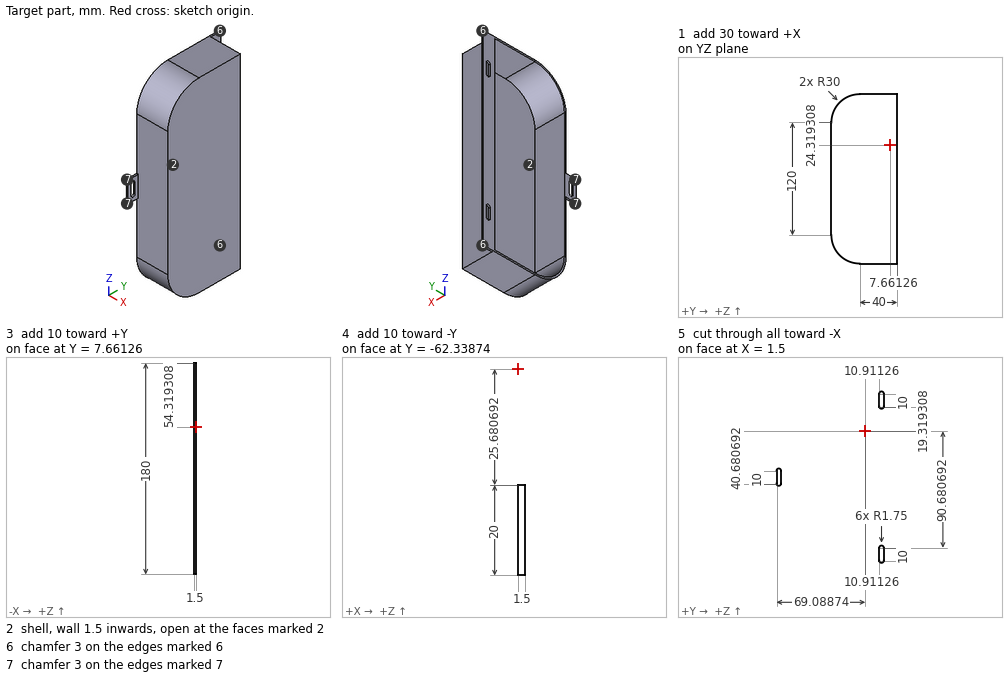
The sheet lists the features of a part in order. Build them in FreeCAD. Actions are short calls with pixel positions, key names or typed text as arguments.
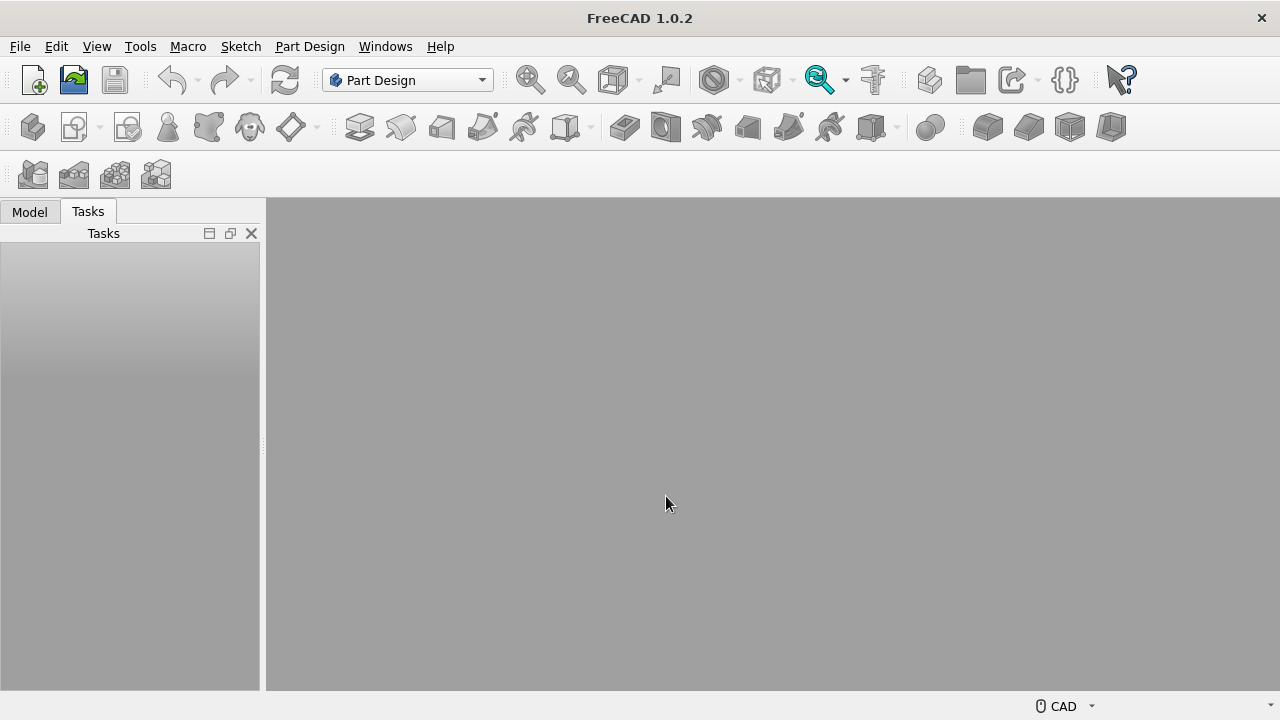
click(33, 80)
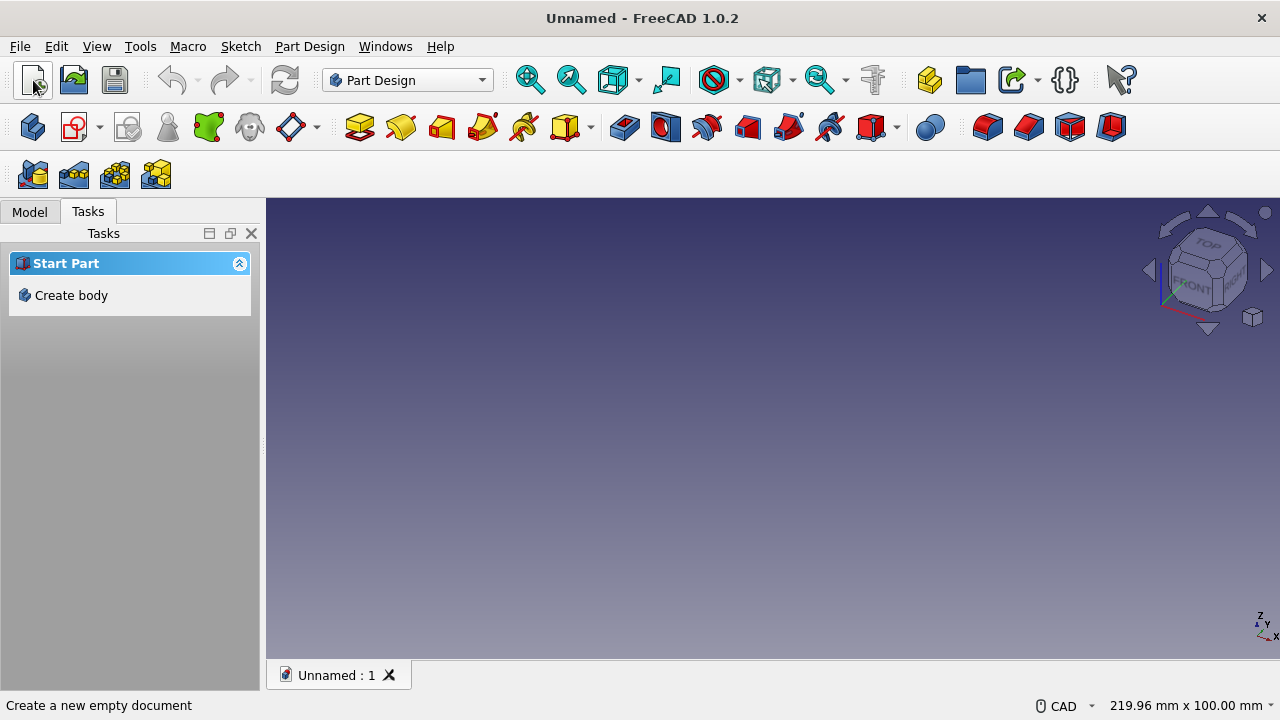
click(74, 128)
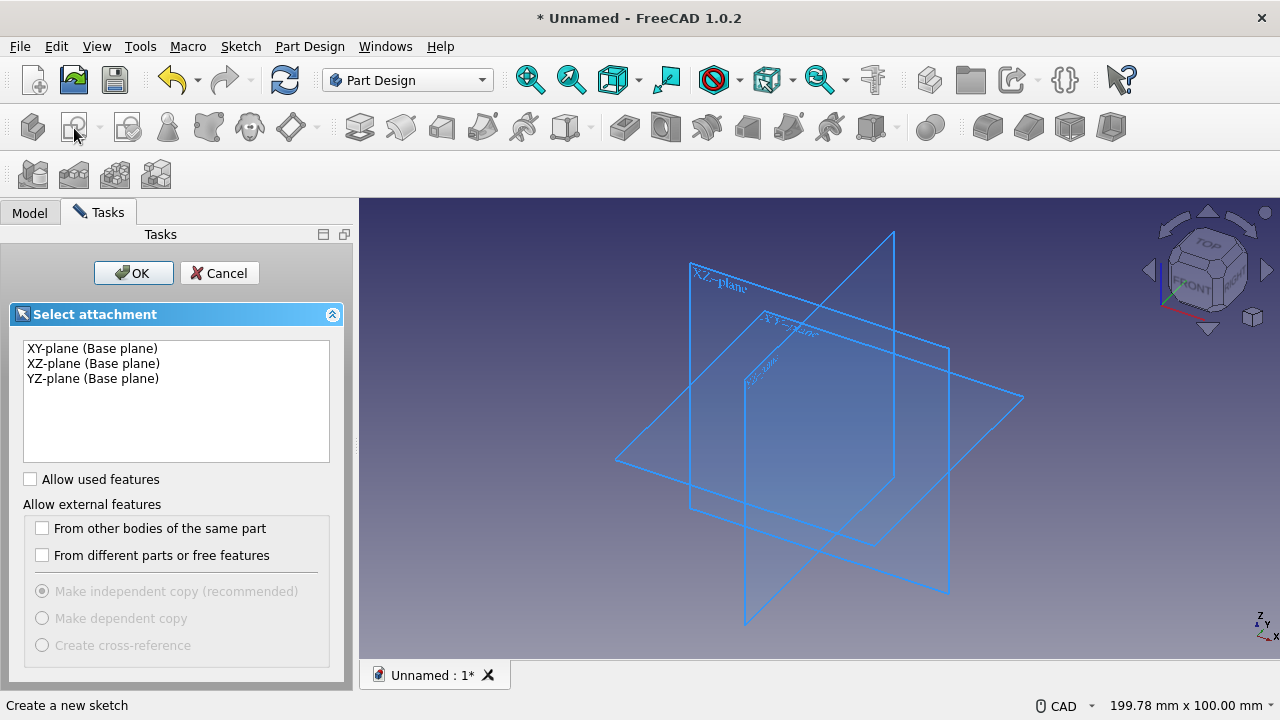
click(84, 378)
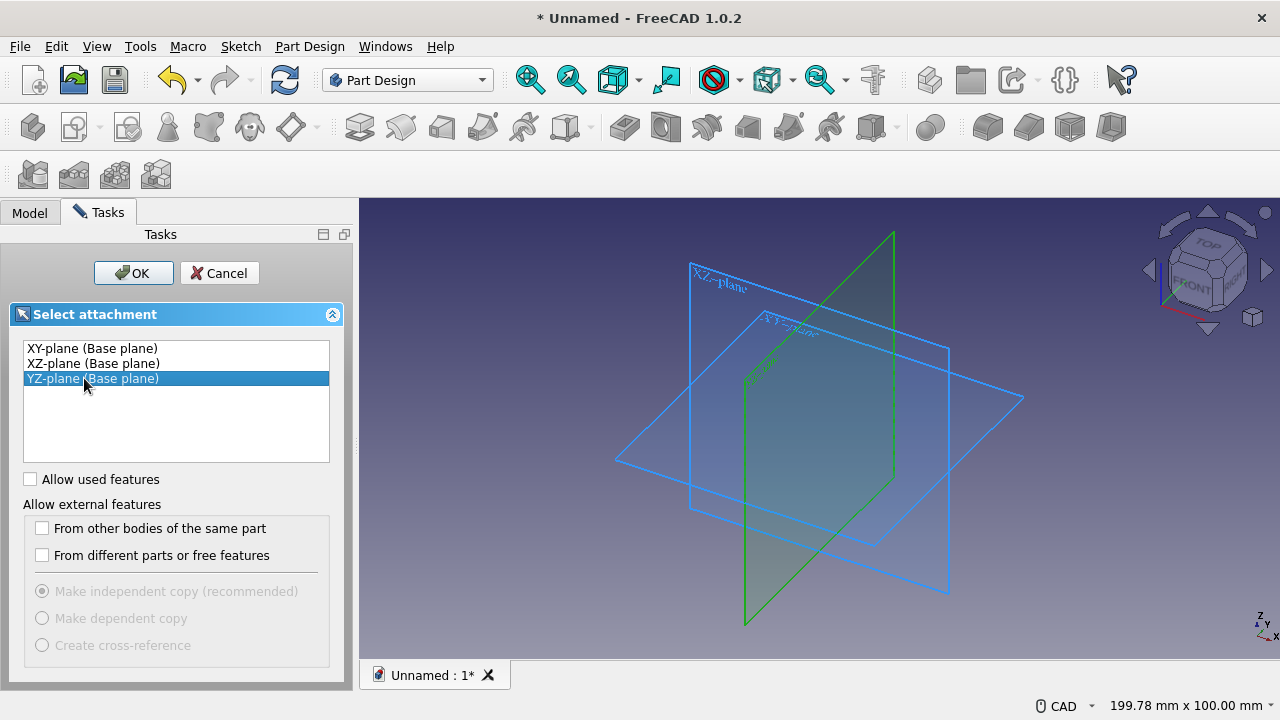
click(134, 273)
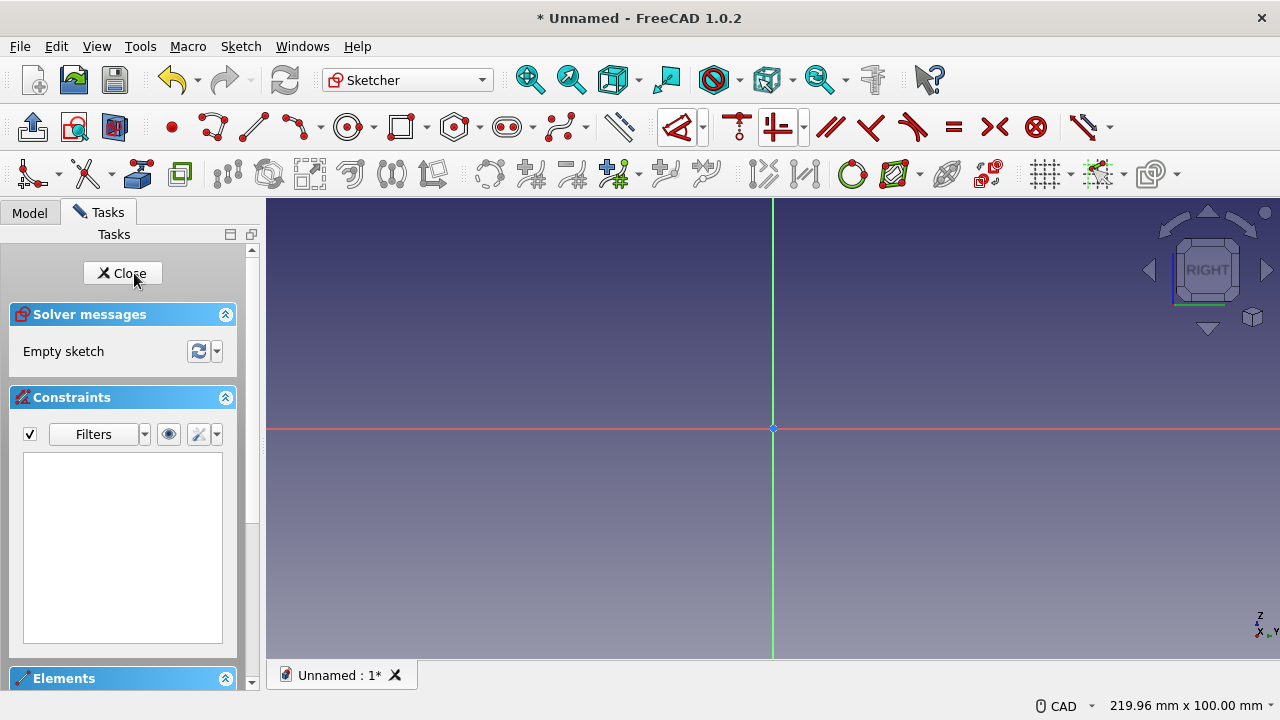
scroll(738, 333, down, 5)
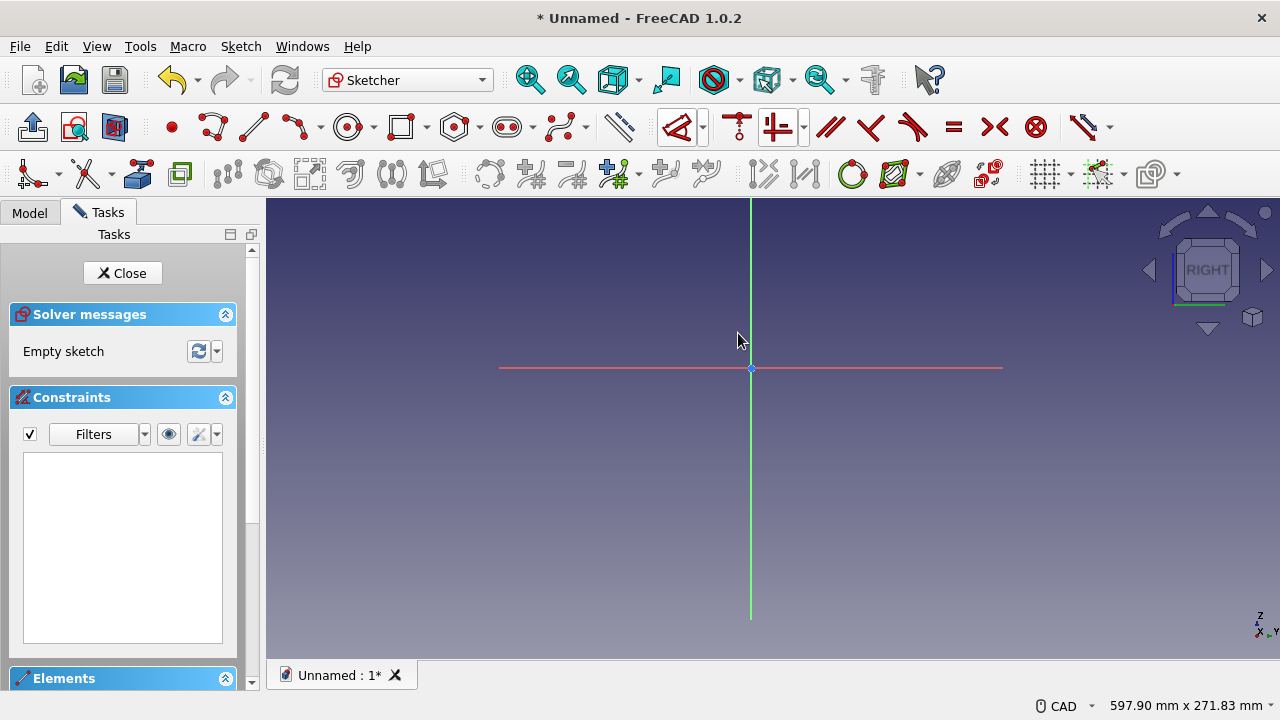
click(254, 128)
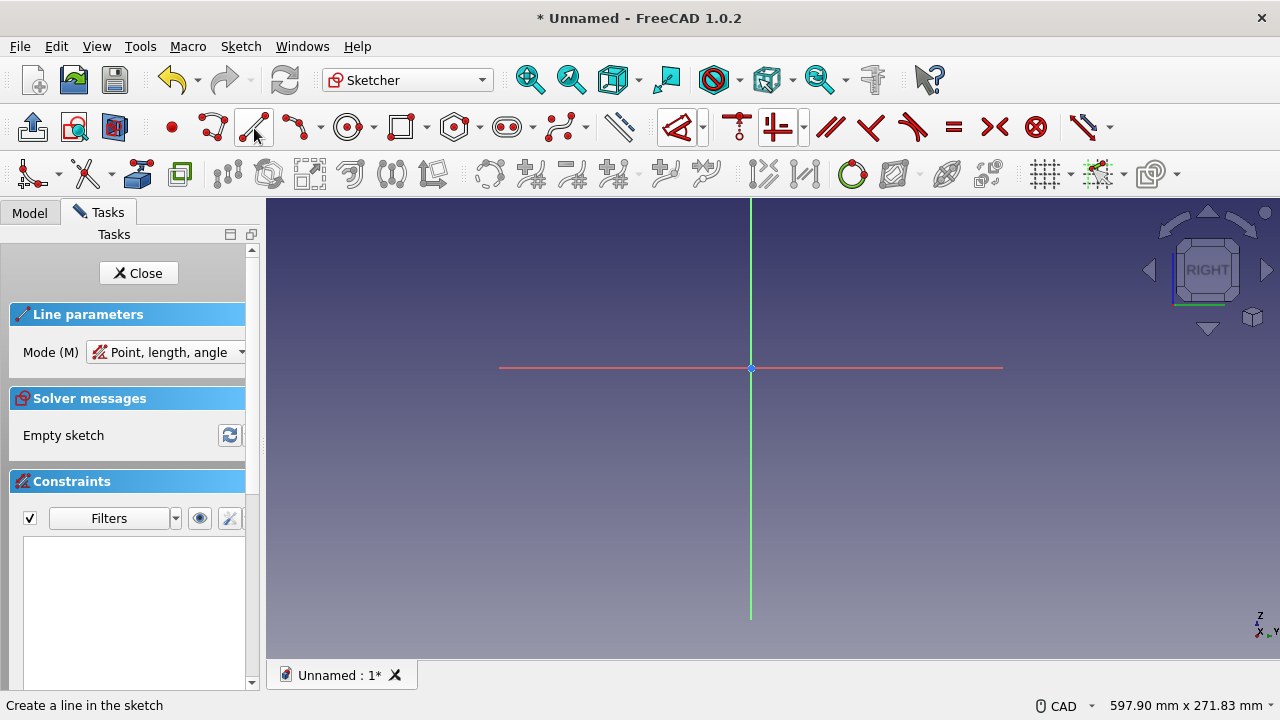
click(645, 327)
click(645, 531)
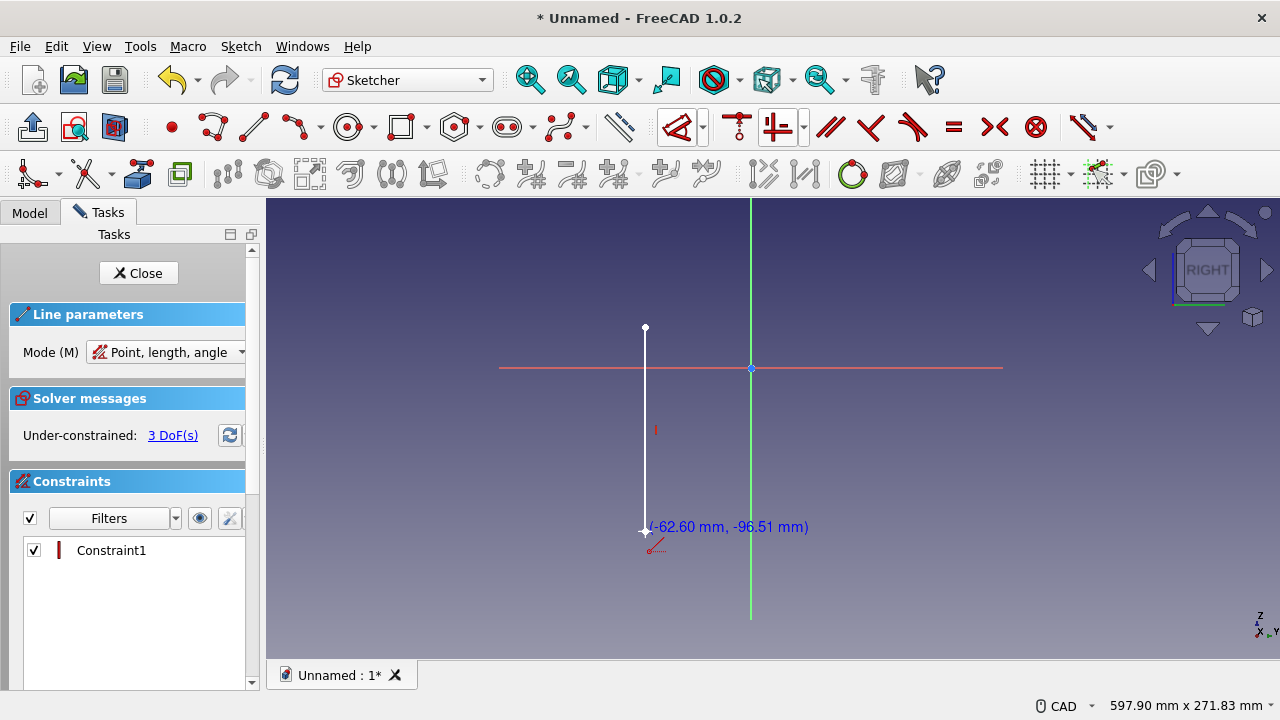
click(213, 128)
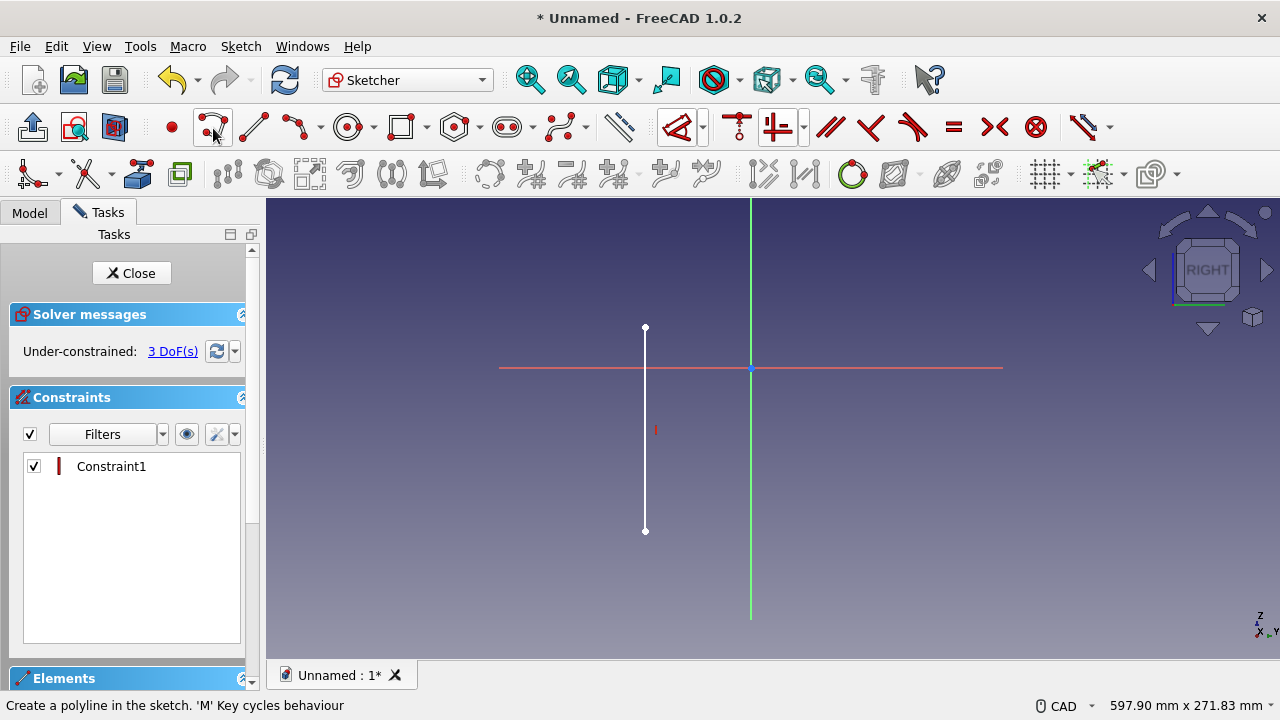
click(696, 581)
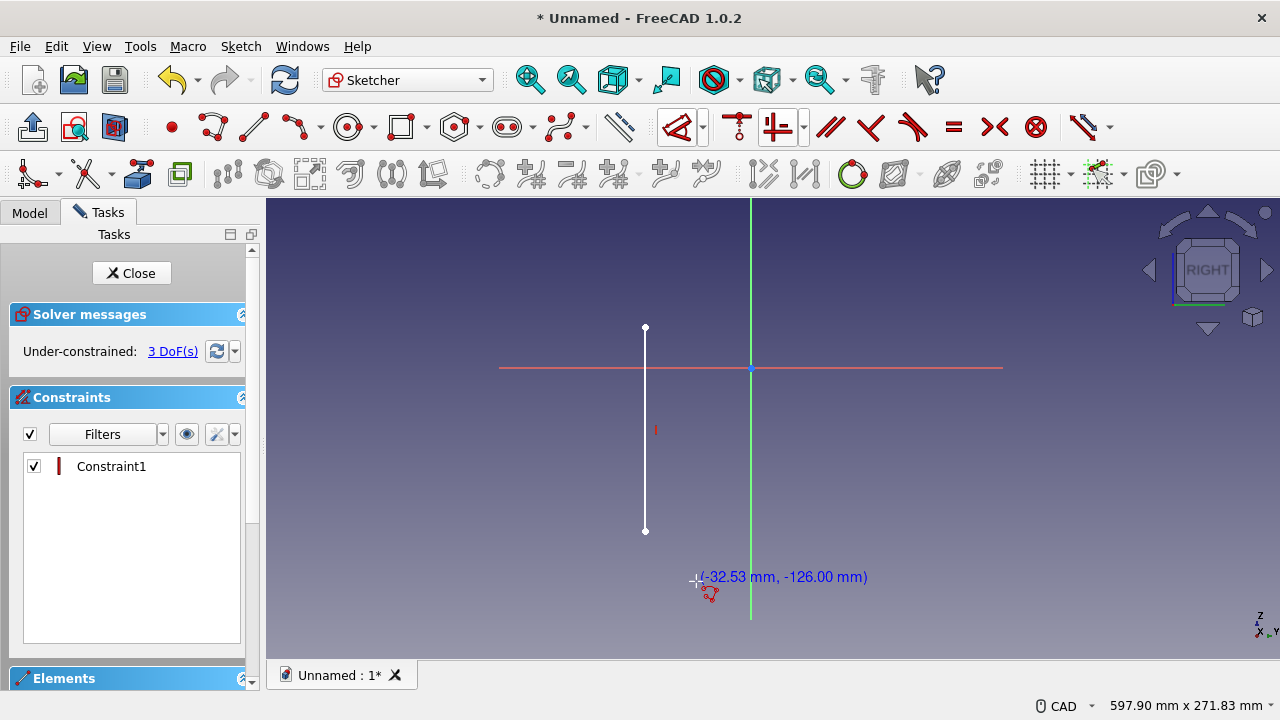
scroll(764, 581, up, 2)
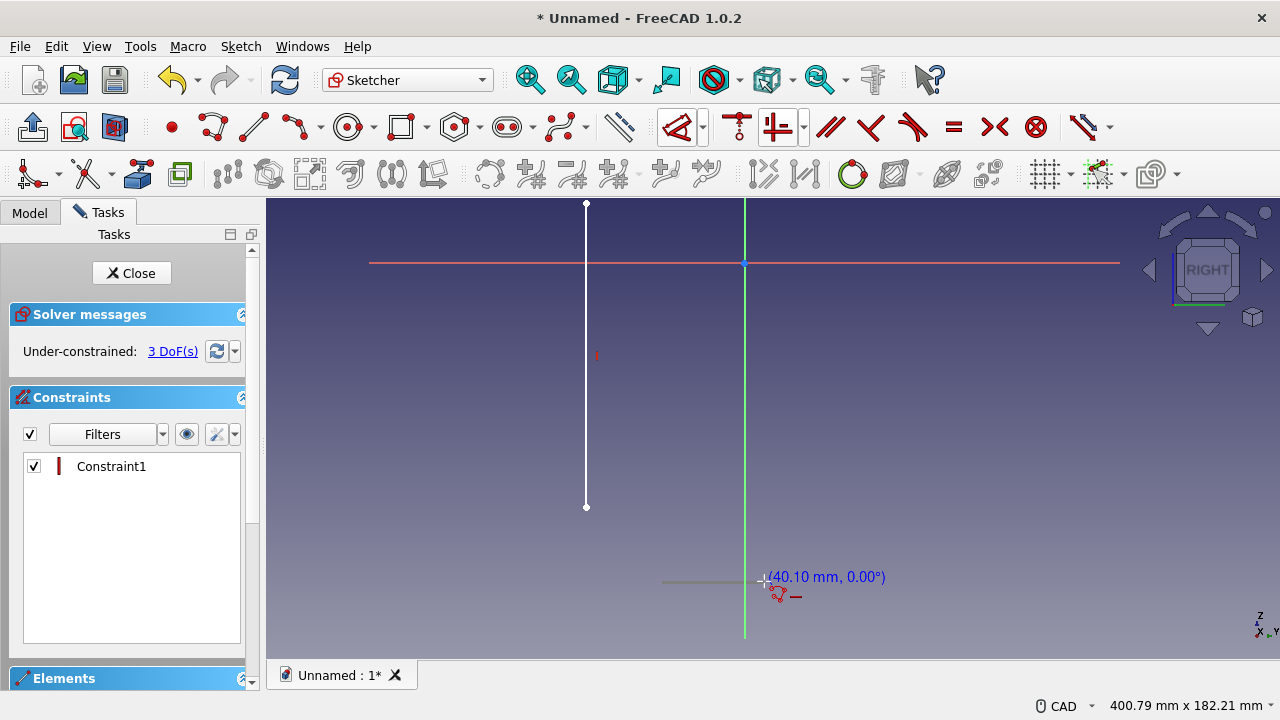
click(764, 581)